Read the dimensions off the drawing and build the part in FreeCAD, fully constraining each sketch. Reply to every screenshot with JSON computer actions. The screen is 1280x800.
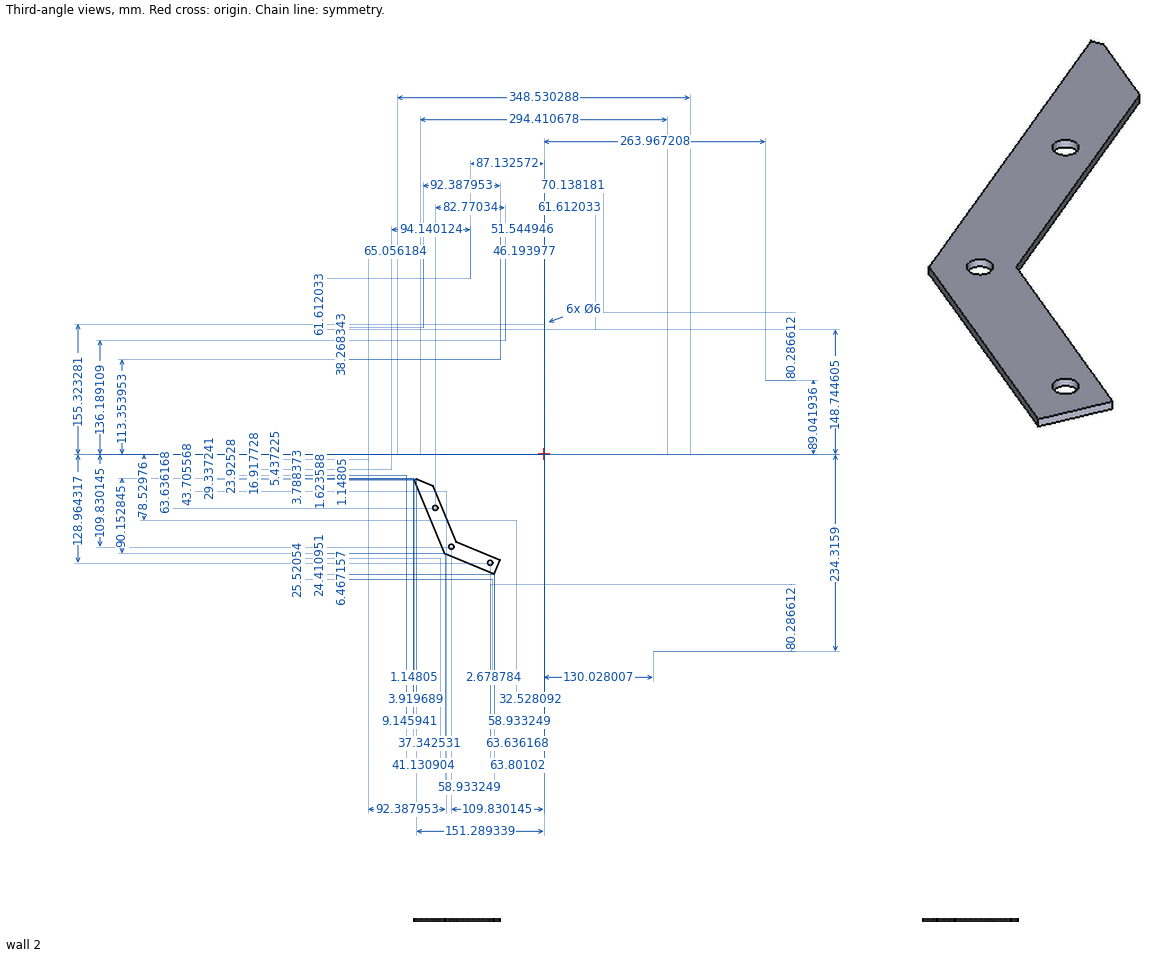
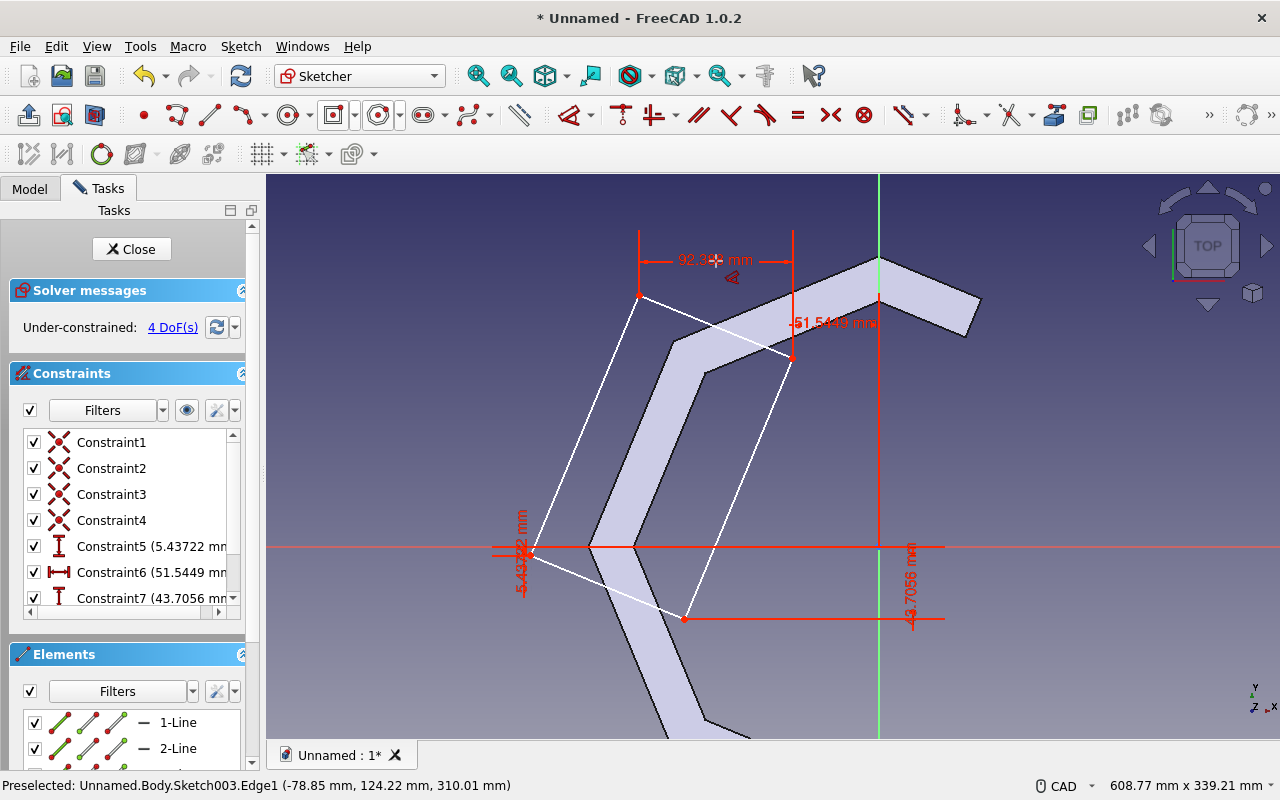
{"action": "left_click", "coordinate": [747, 340]}
{"action": "left_click", "coordinate": [827, 349]}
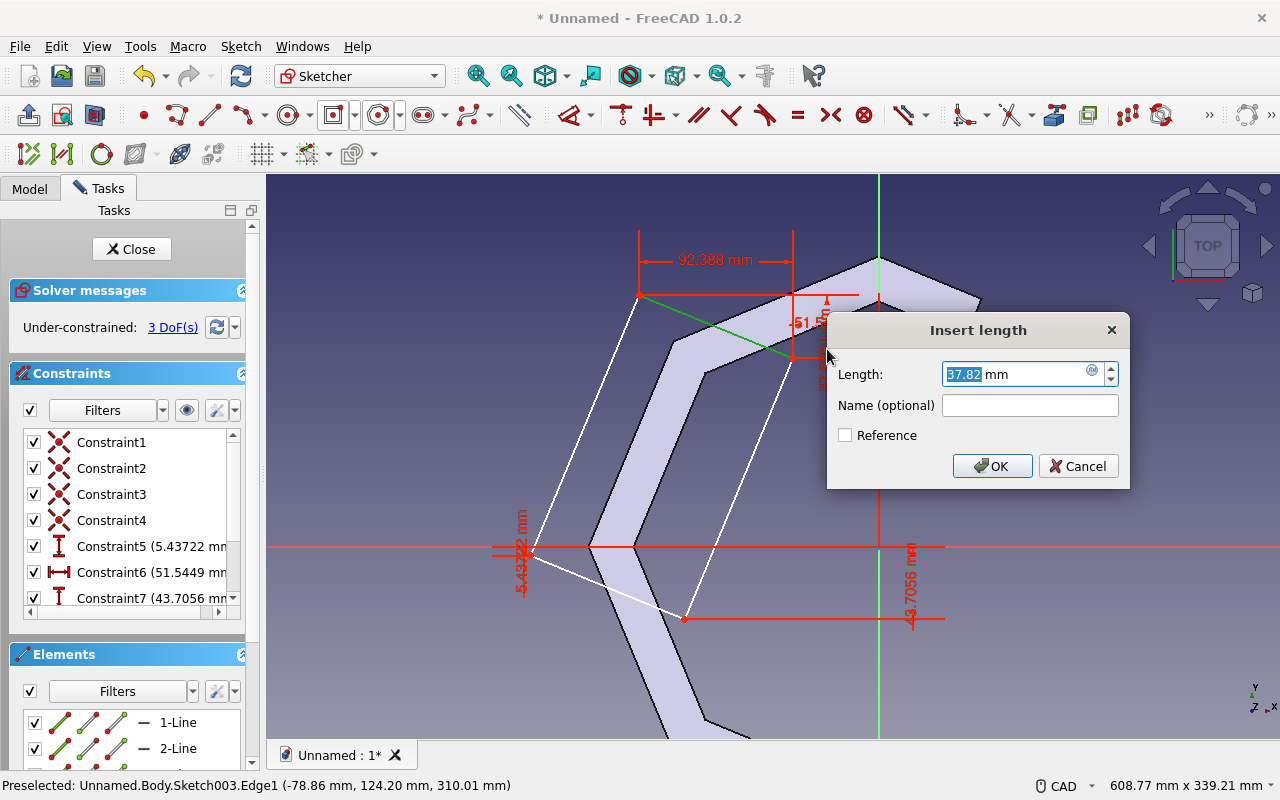
{"action": "type", "text": "38.268343"}
{"action": "key", "text": "Return"}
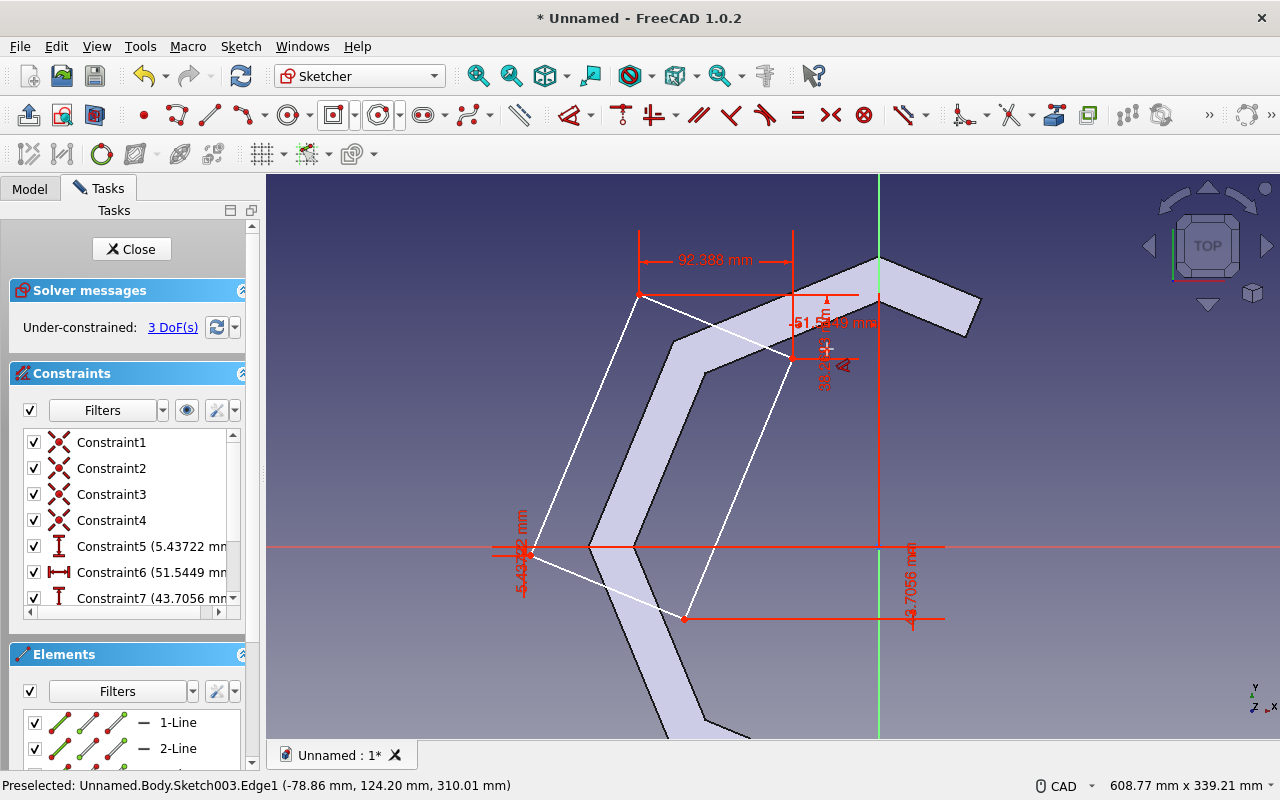
{"action": "left_click", "coordinate": [607, 373]}
{"action": "left_click", "coordinate": [585, 261]}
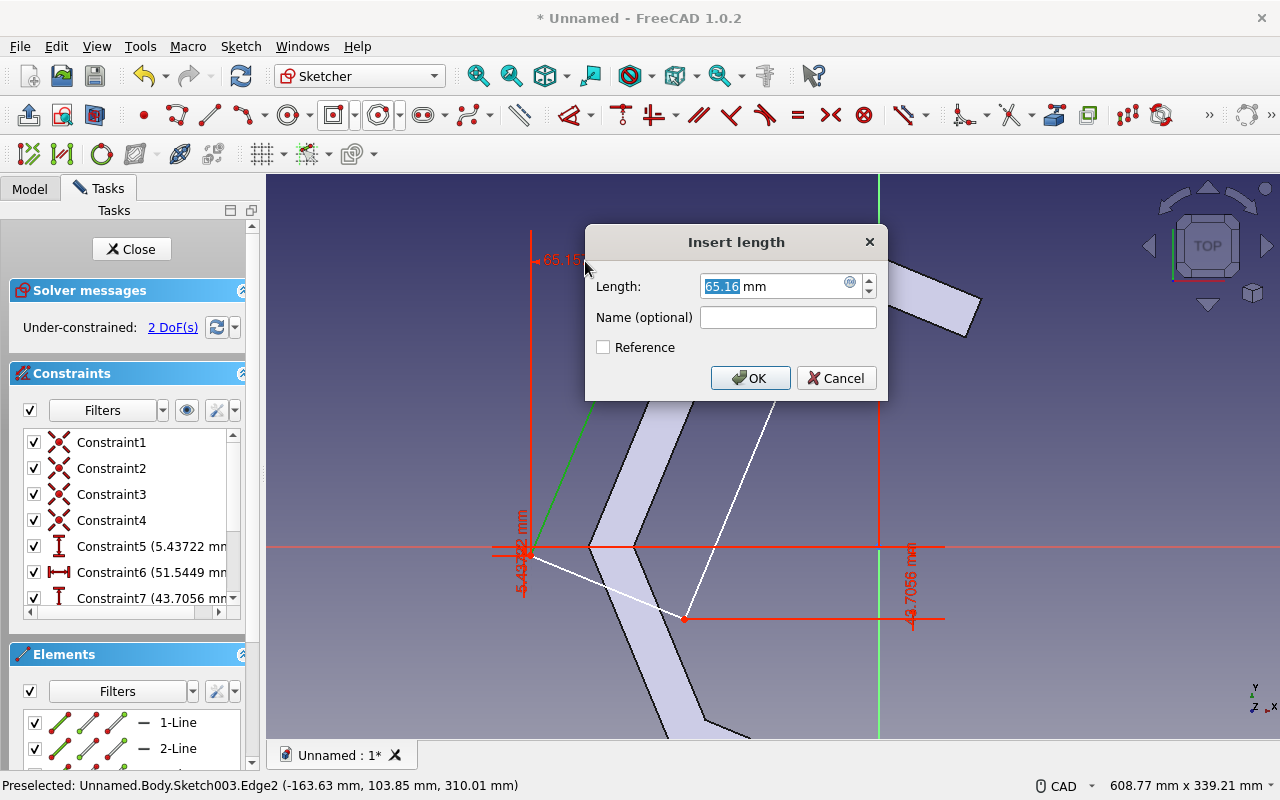
{"action": "type", "text": "65.056184"}
{"action": "key", "text": "Return"}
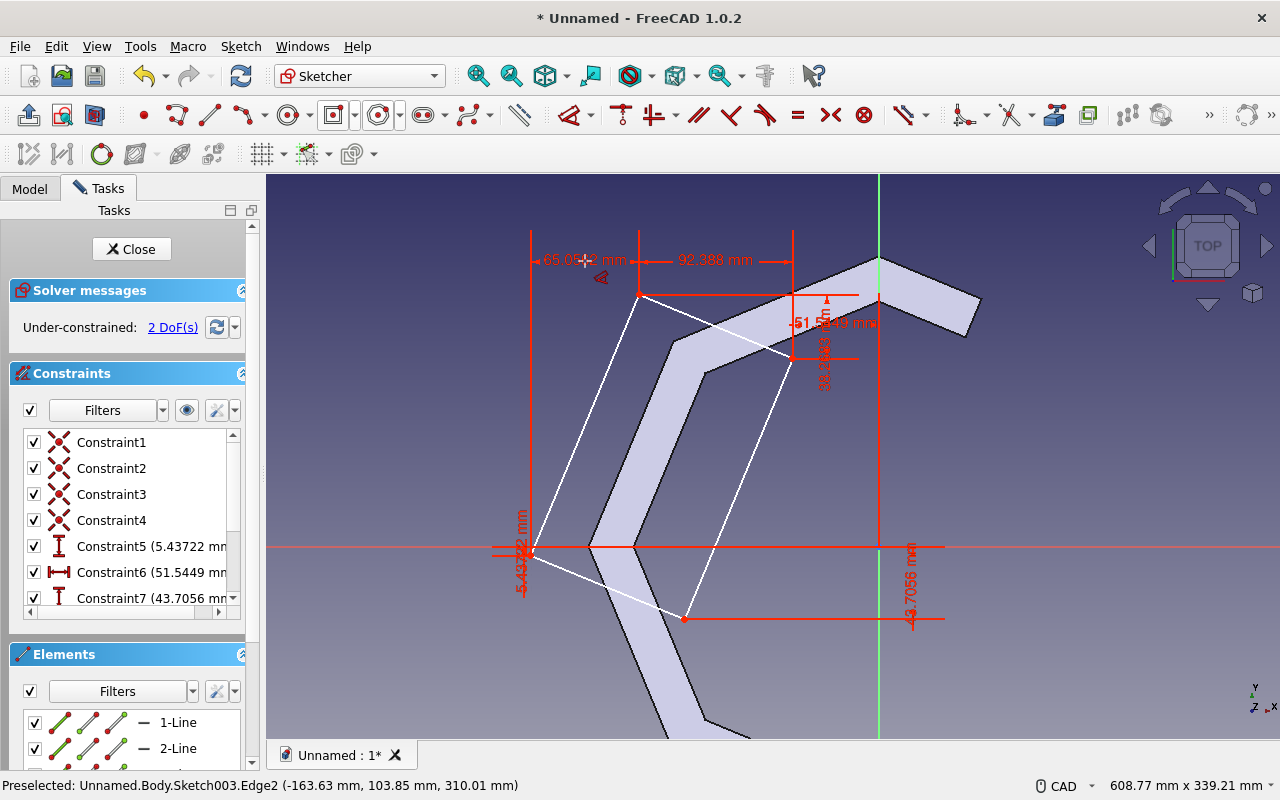
{"action": "left_click", "coordinate": [577, 575]}
{"action": "left_click", "coordinate": [608, 653]}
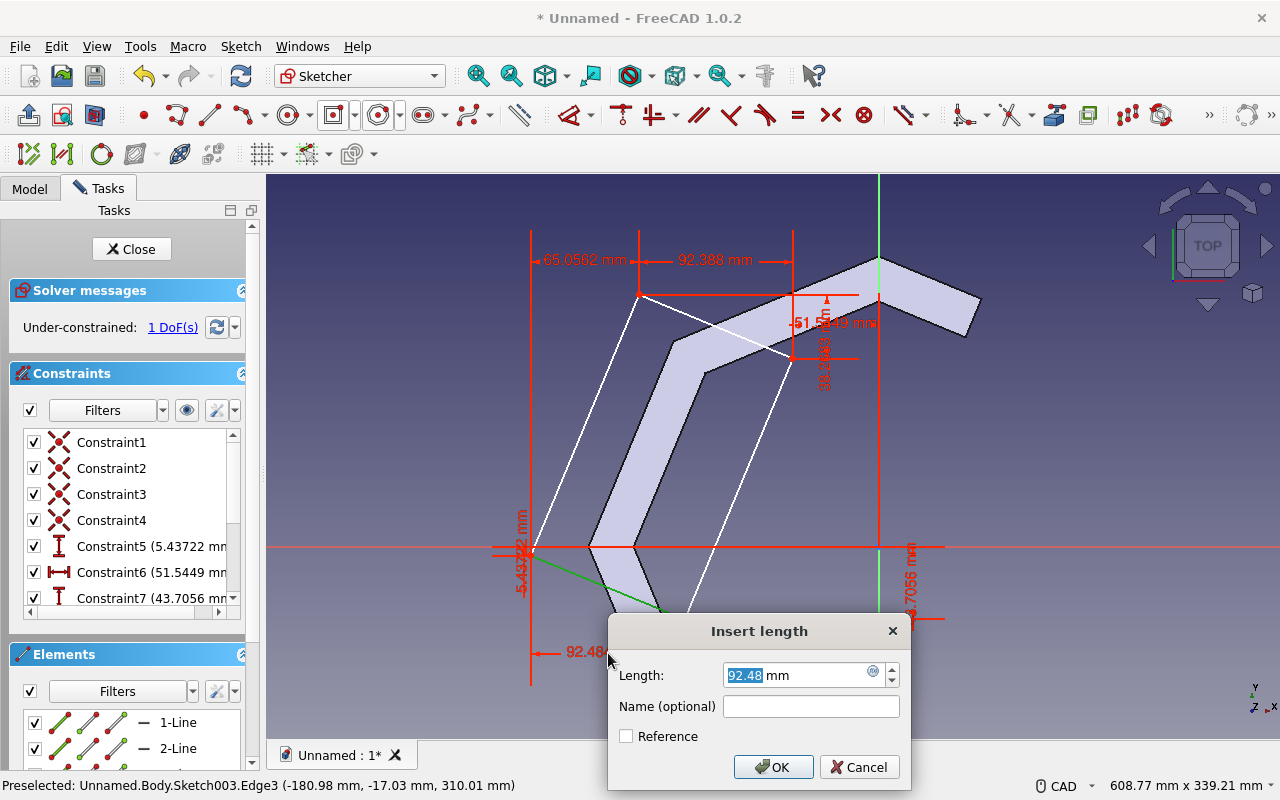
{"action": "type", "text": "92.387953"}
{"action": "key", "text": "Return"}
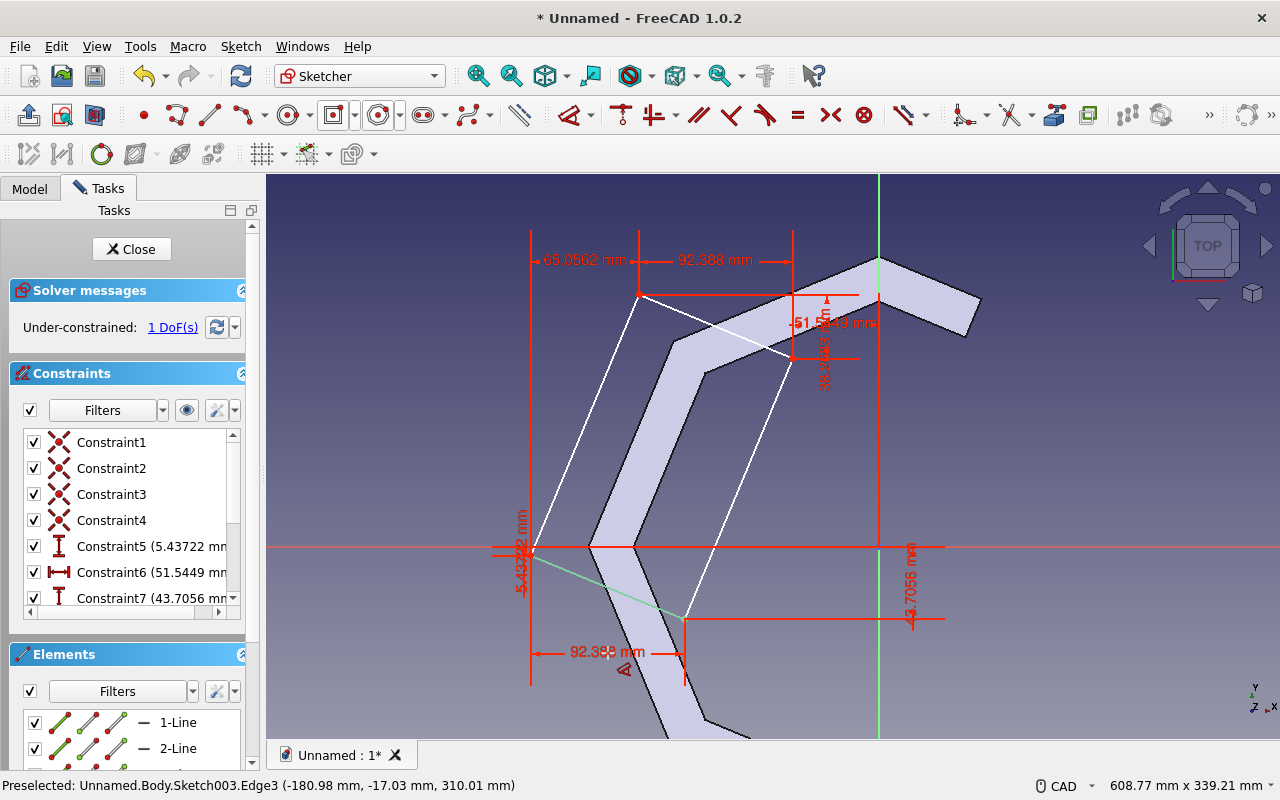
{"action": "left_click", "coordinate": [793, 359]}
{"action": "left_click", "coordinate": [913, 453]}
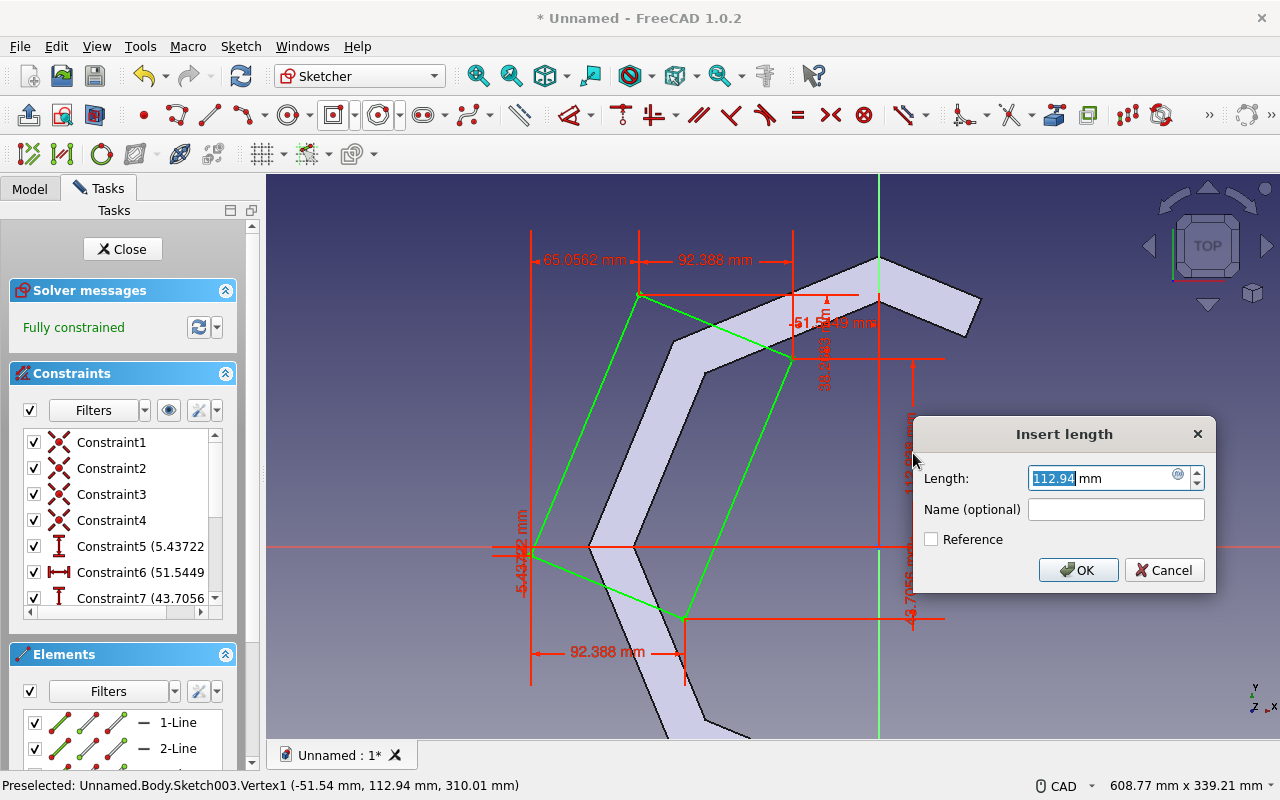
{"action": "type", "text": "113.353953"}
{"action": "key", "text": "Return"}
{"action": "key", "text": "Escape"}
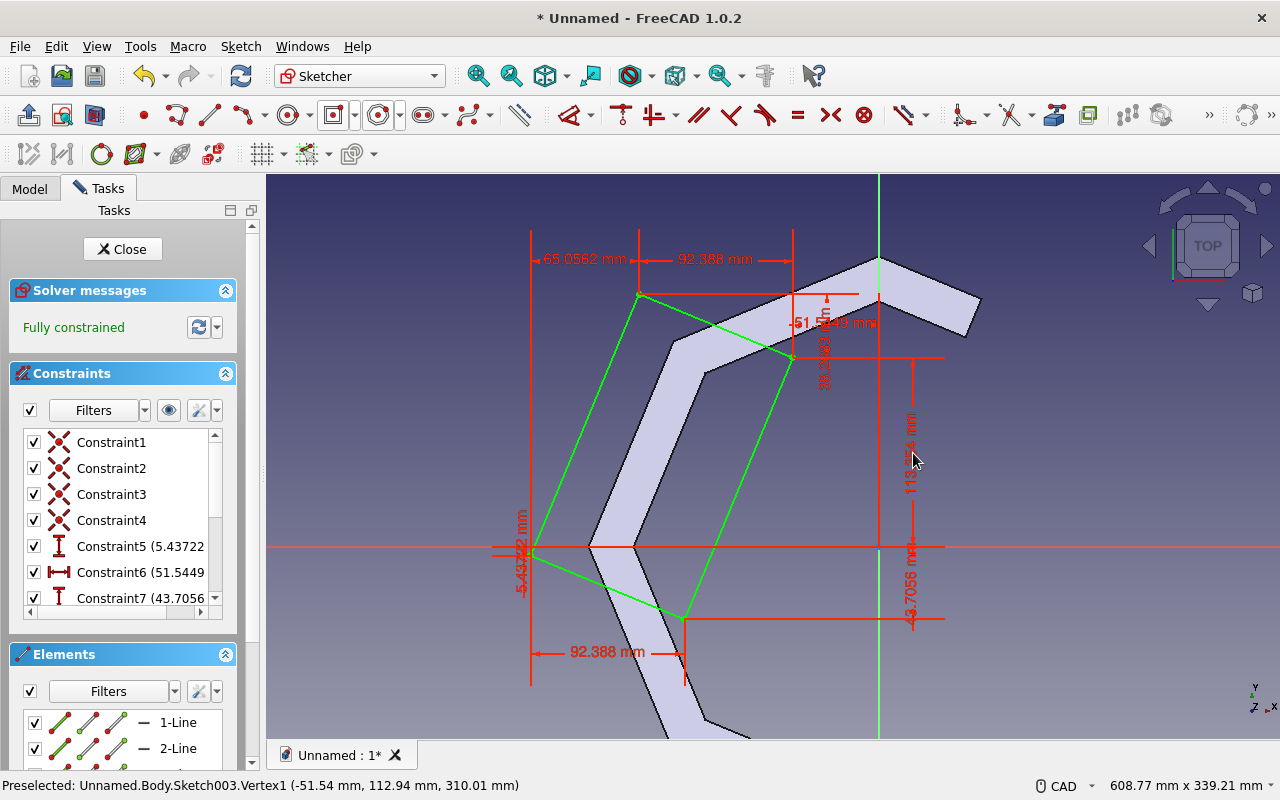
{"action": "left_click", "coordinate": [123, 249]}